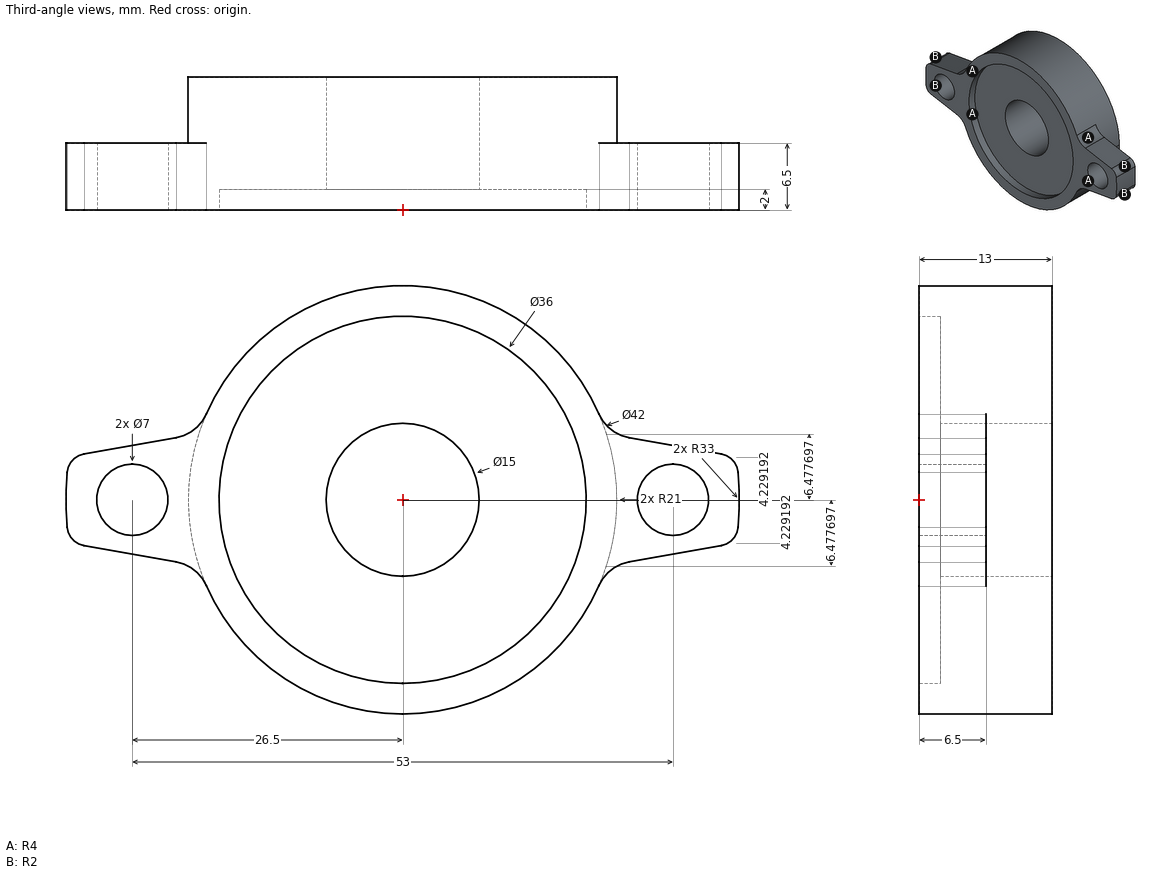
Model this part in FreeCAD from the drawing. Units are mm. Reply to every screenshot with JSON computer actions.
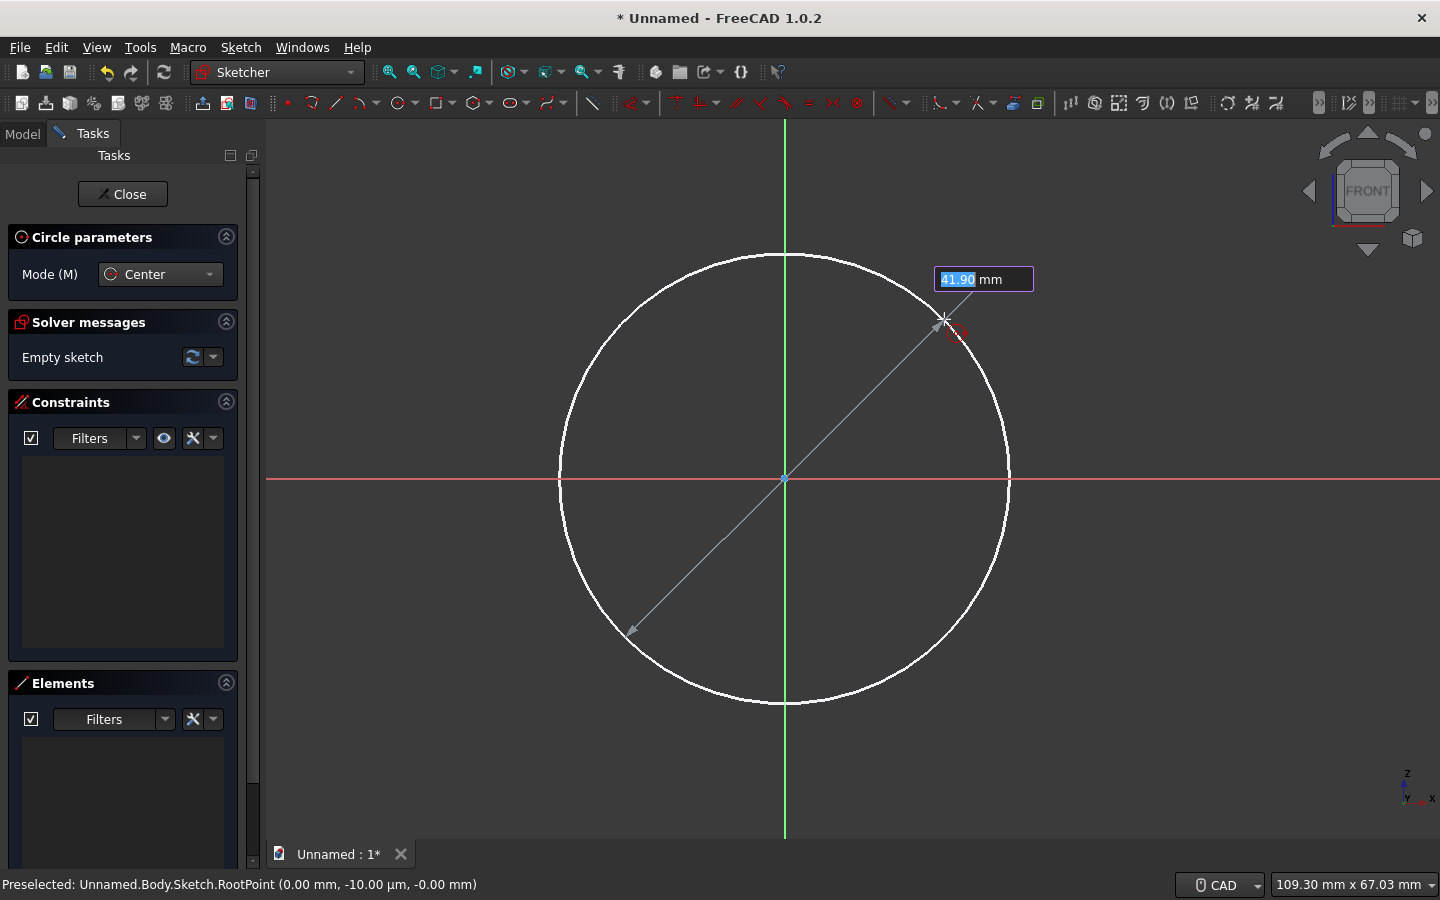
{"action": "type", "text": "42"}
{"action": "key", "text": "Return"}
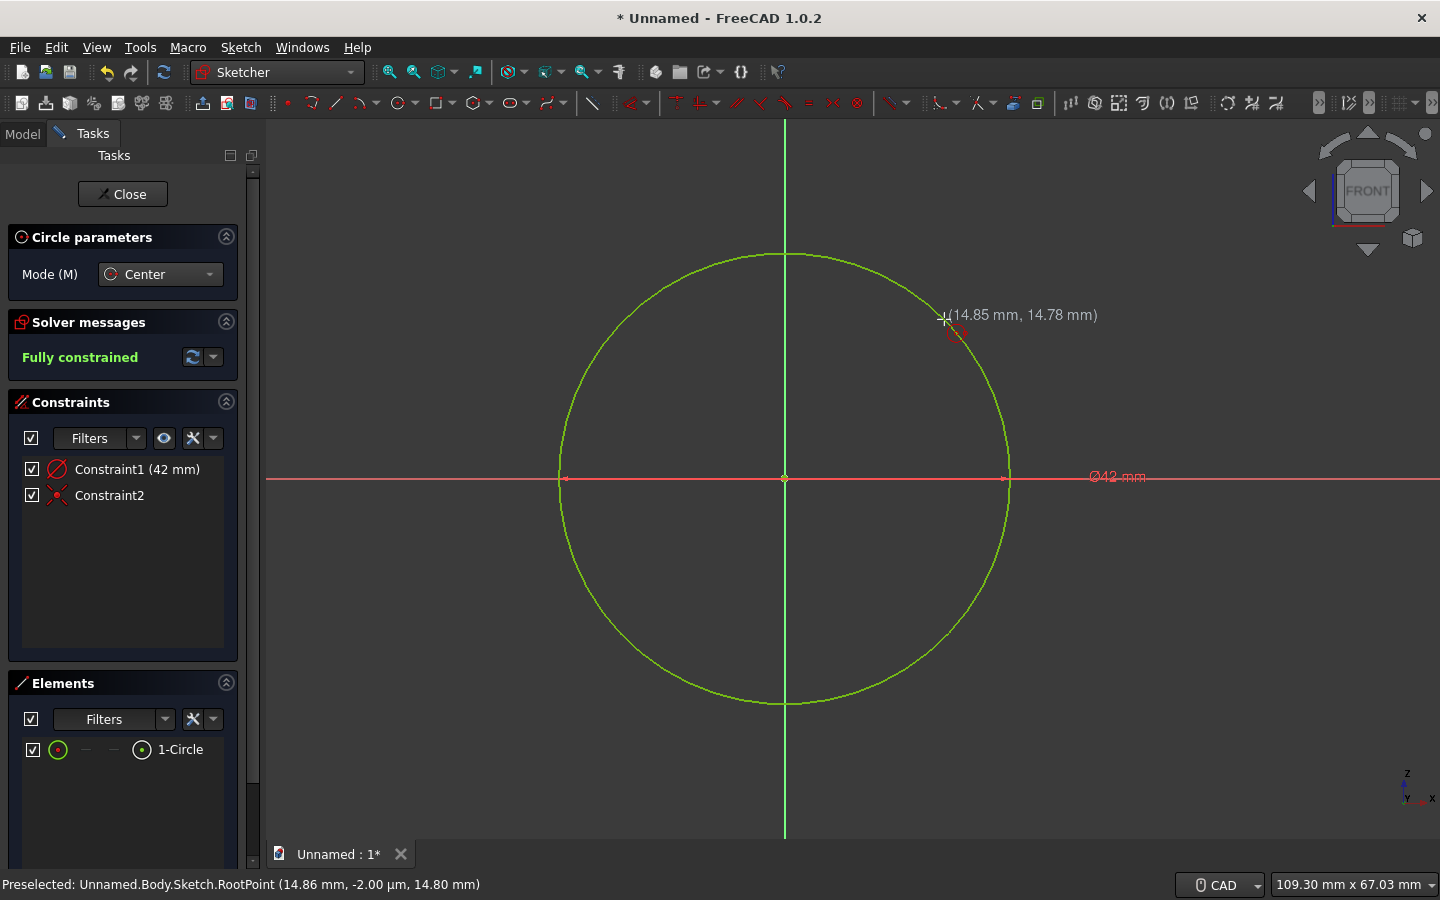
{"action": "left_click", "coordinate": [785, 479]}
{"action": "mouse_move", "coordinate": [841, 422]}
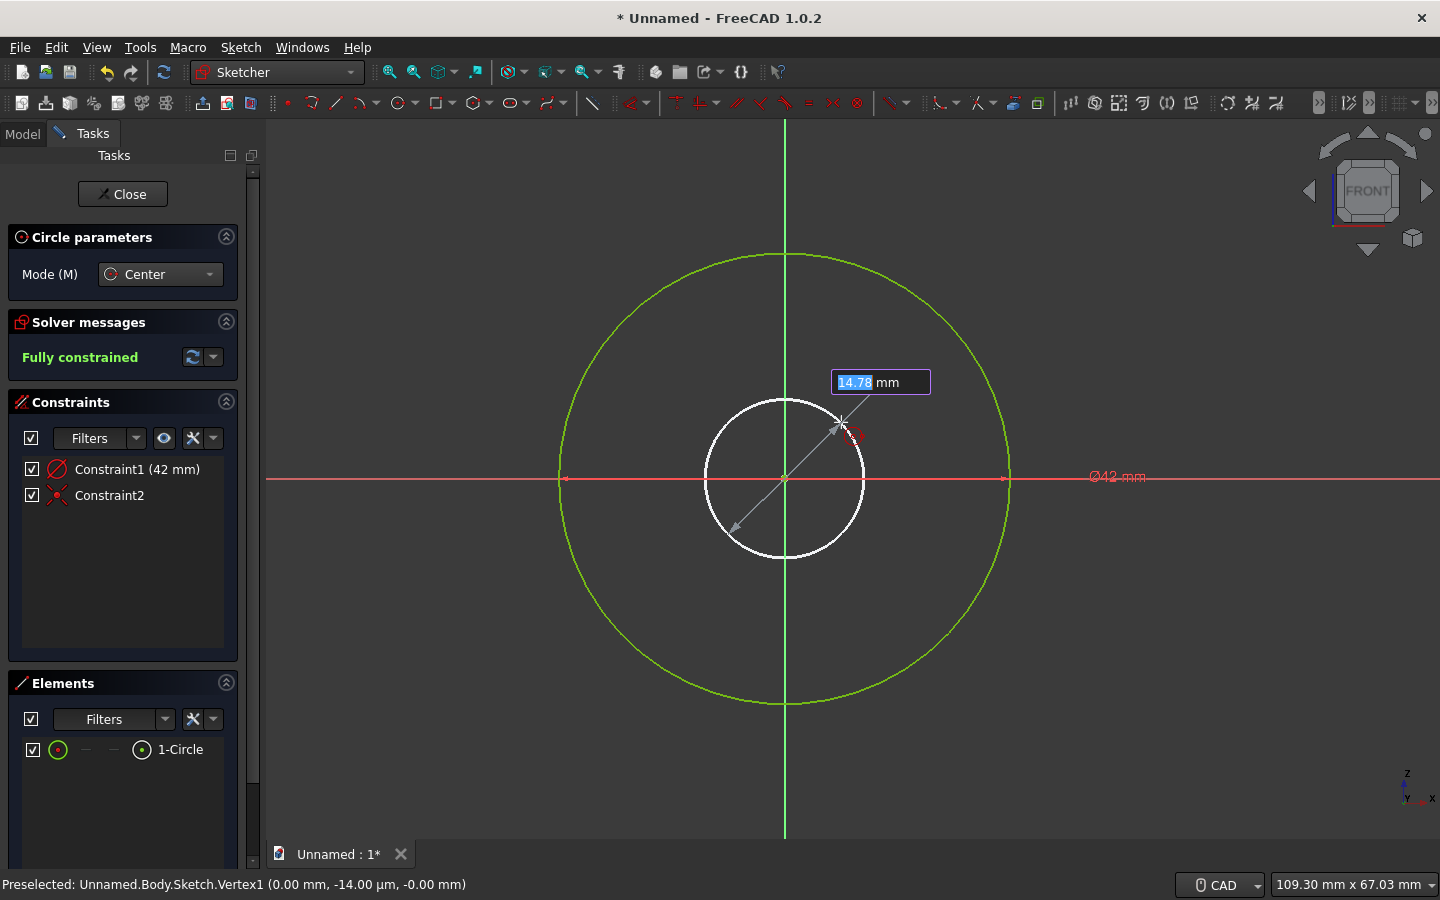
{"action": "type", "text": "15"}
{"action": "key", "text": "Return"}
{"action": "key", "text": "Escape"}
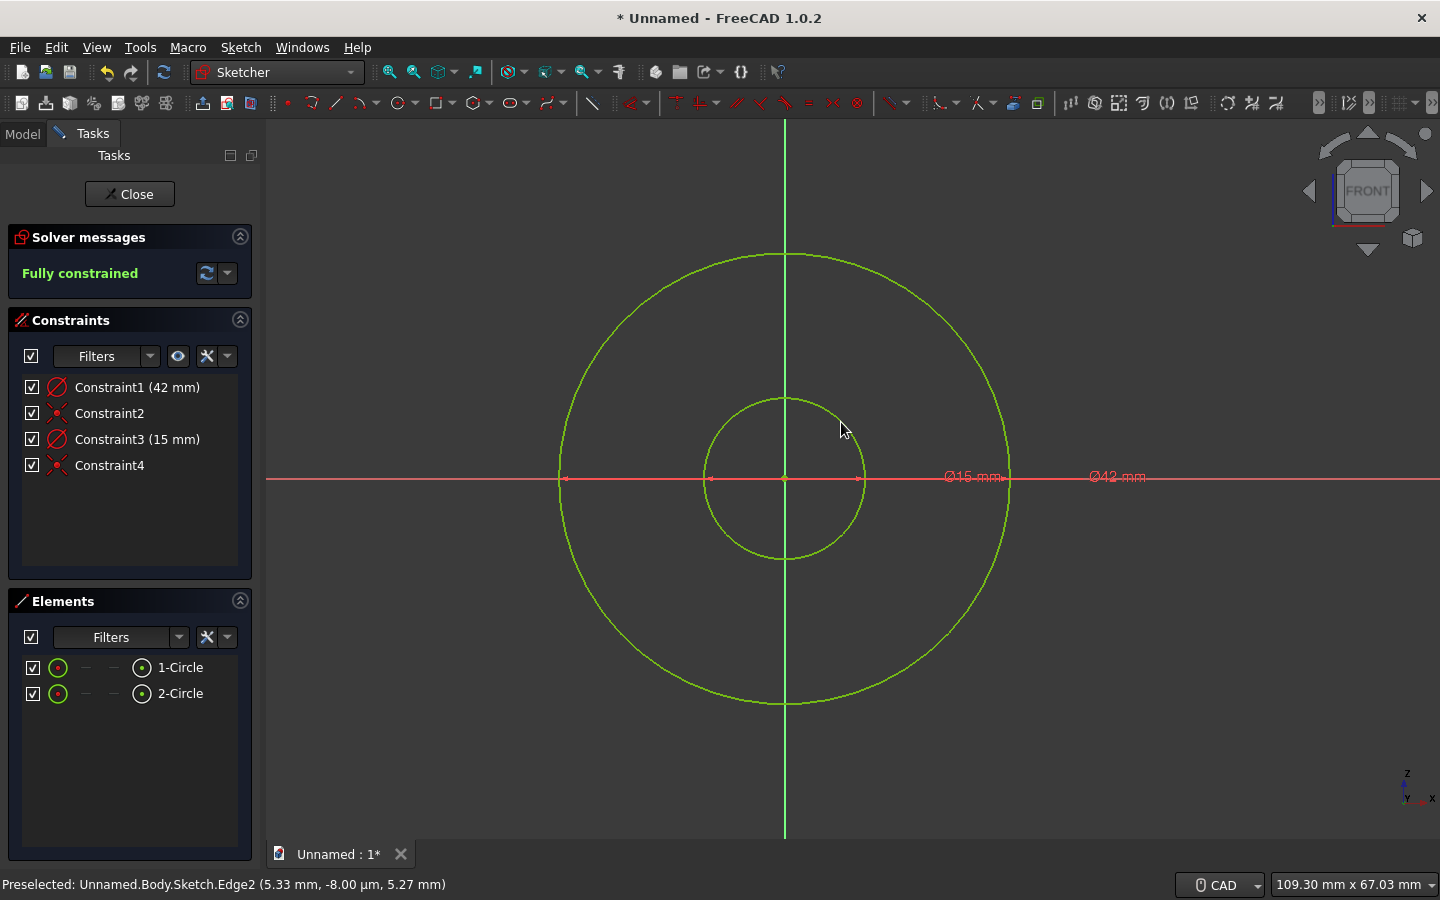
{"action": "left_click", "coordinate": [130, 194]}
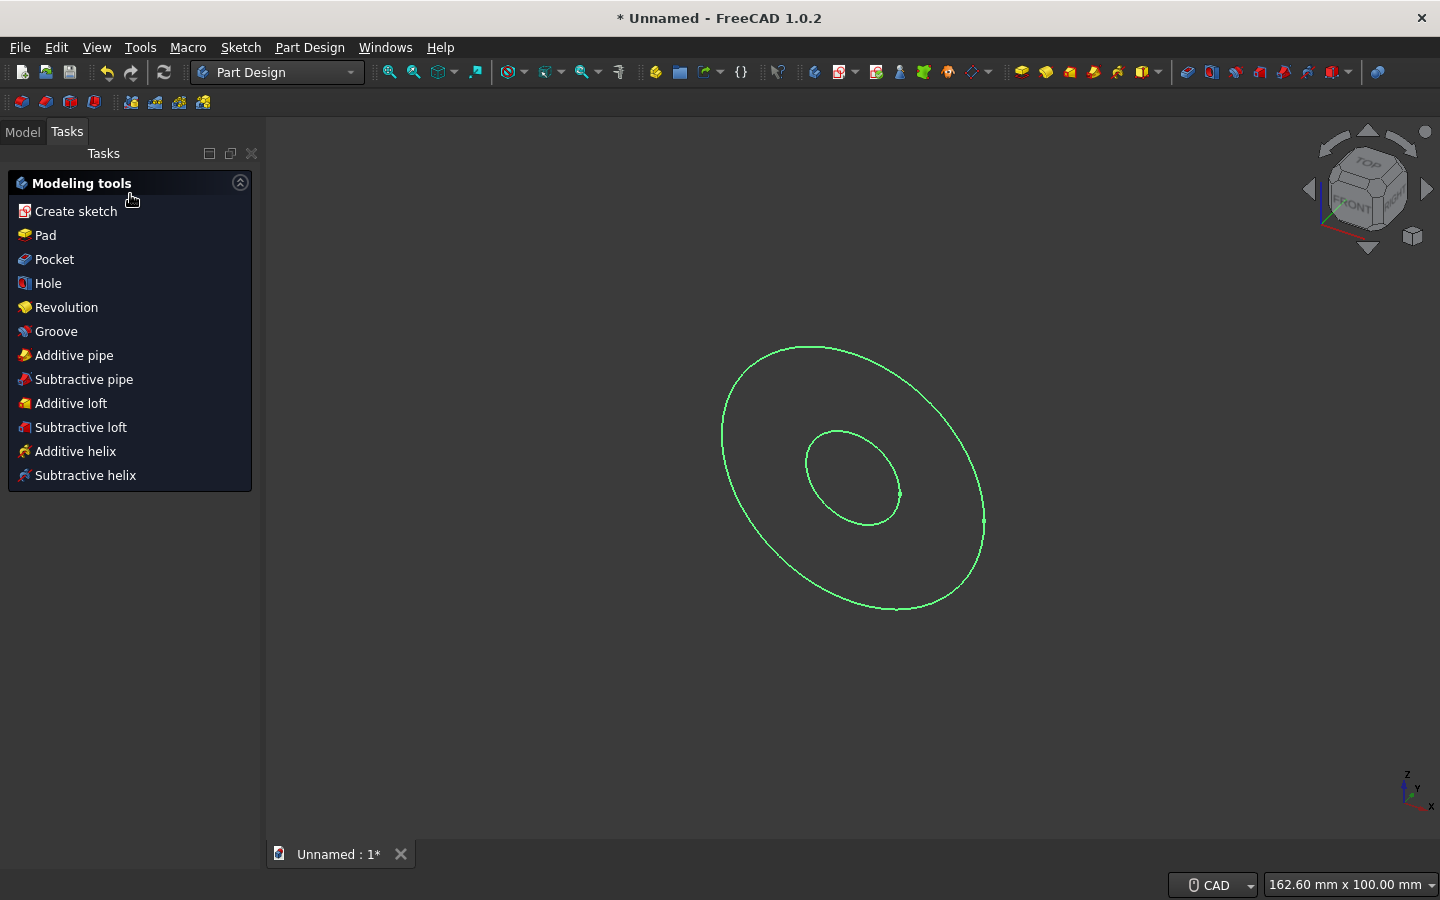
{"action": "left_click", "coordinate": [1022, 72]}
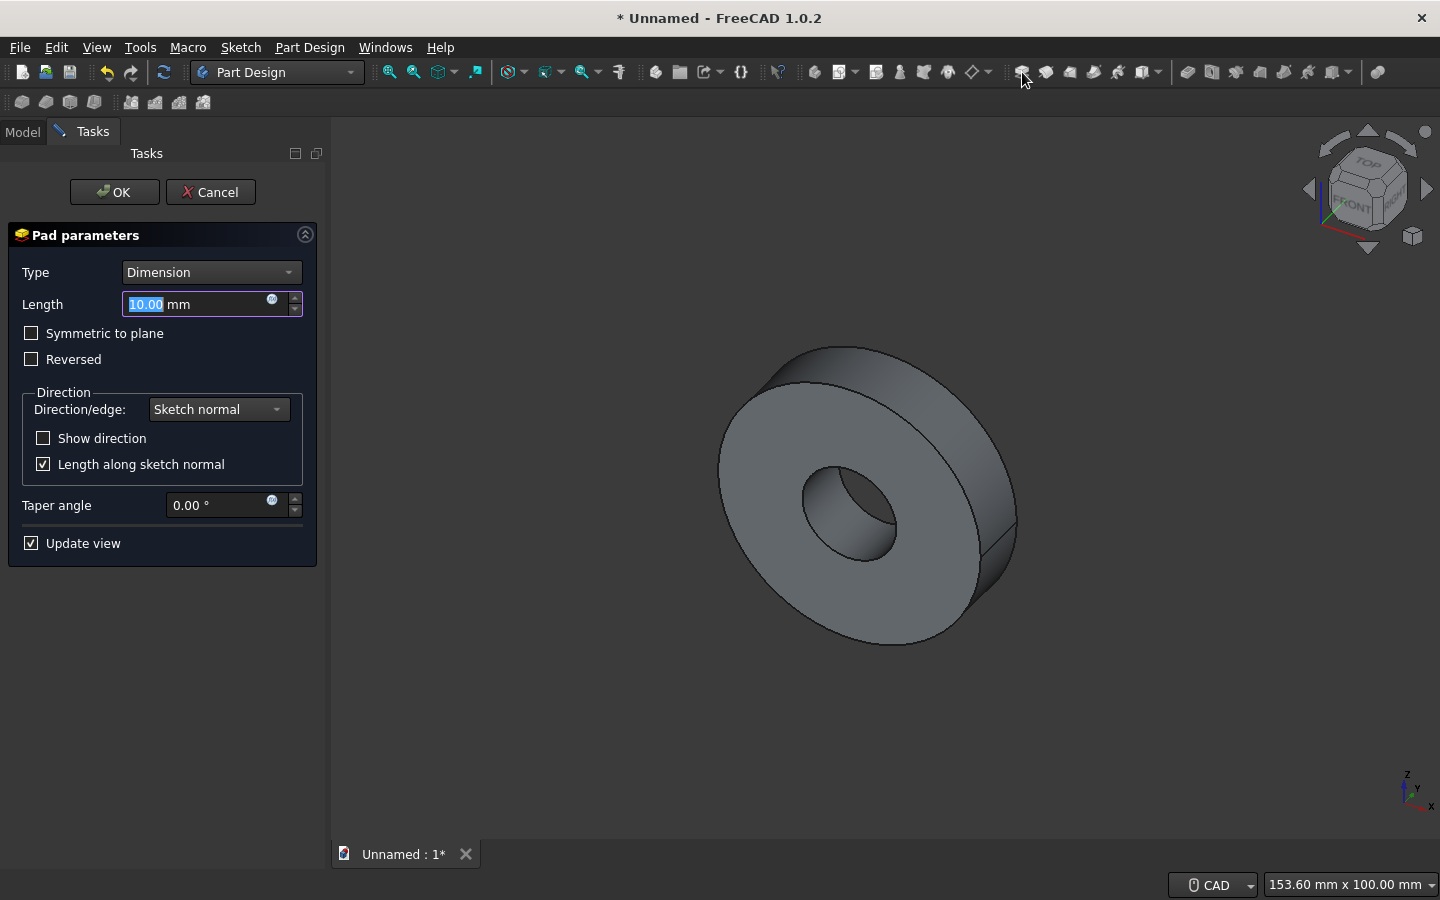
{"action": "type", "text": "13"}
{"action": "key", "text": "Tab"}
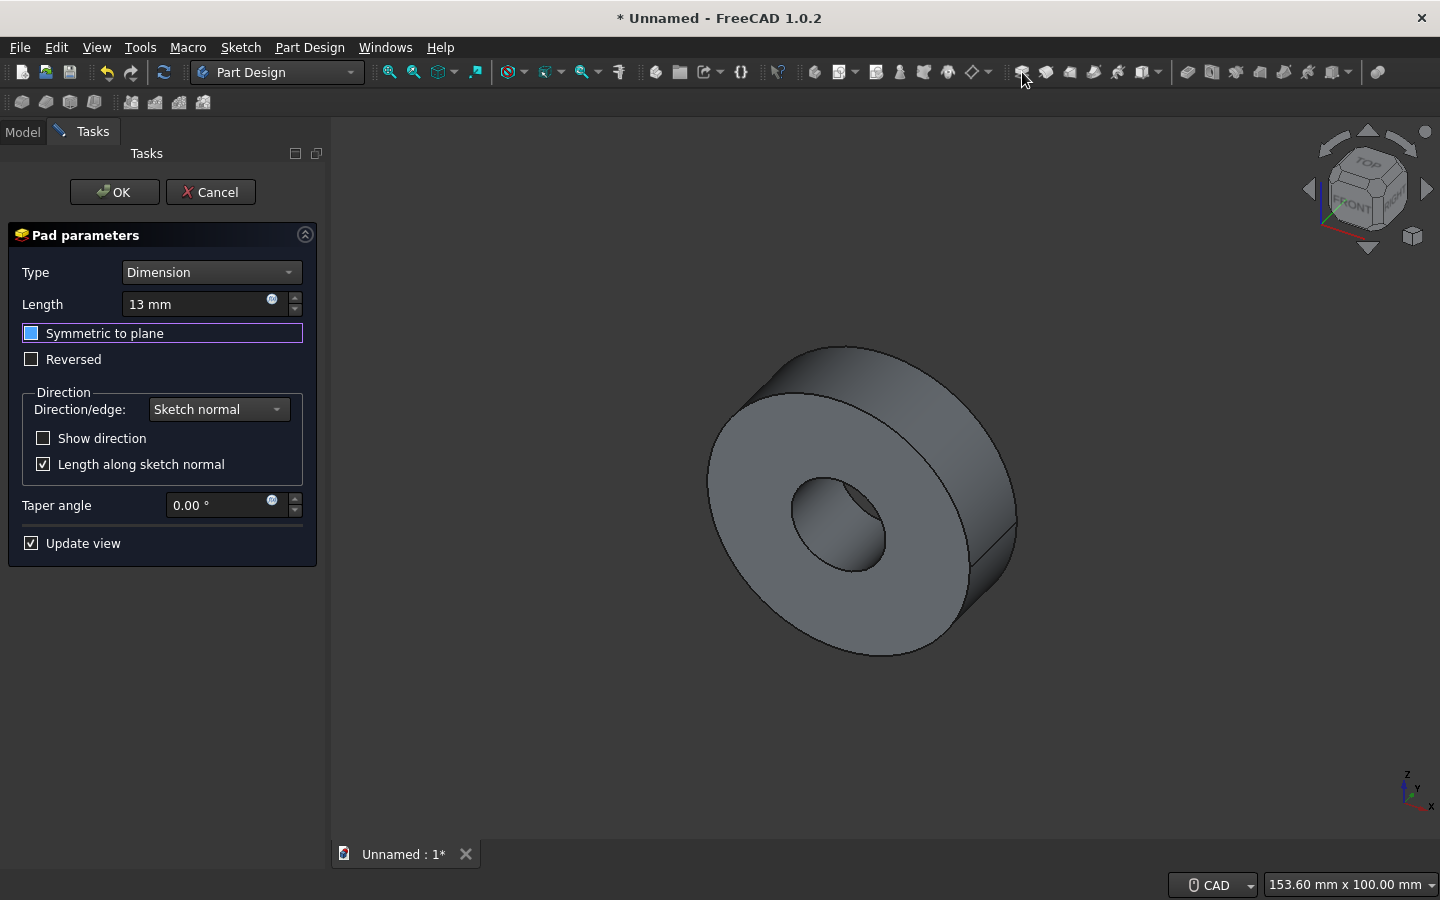
{"action": "left_click", "coordinate": [30, 359]}